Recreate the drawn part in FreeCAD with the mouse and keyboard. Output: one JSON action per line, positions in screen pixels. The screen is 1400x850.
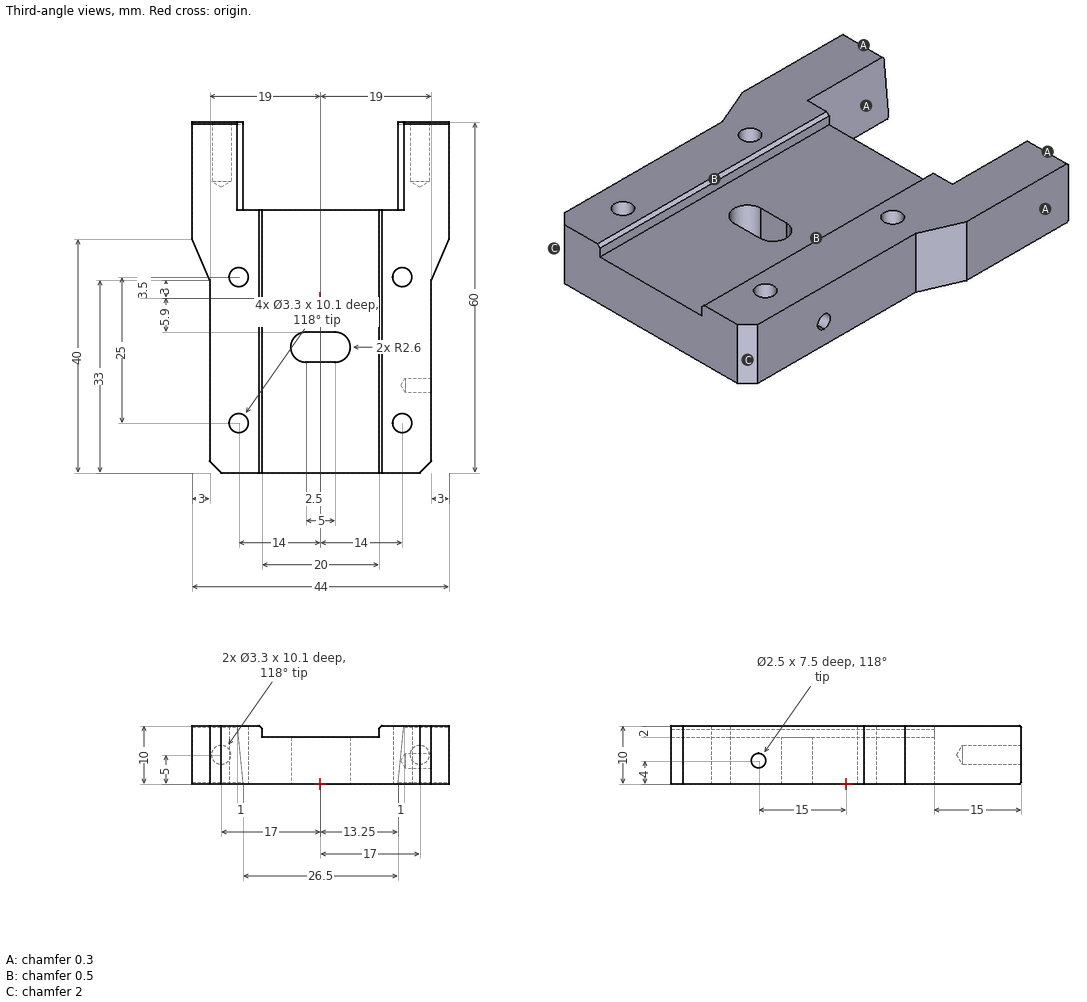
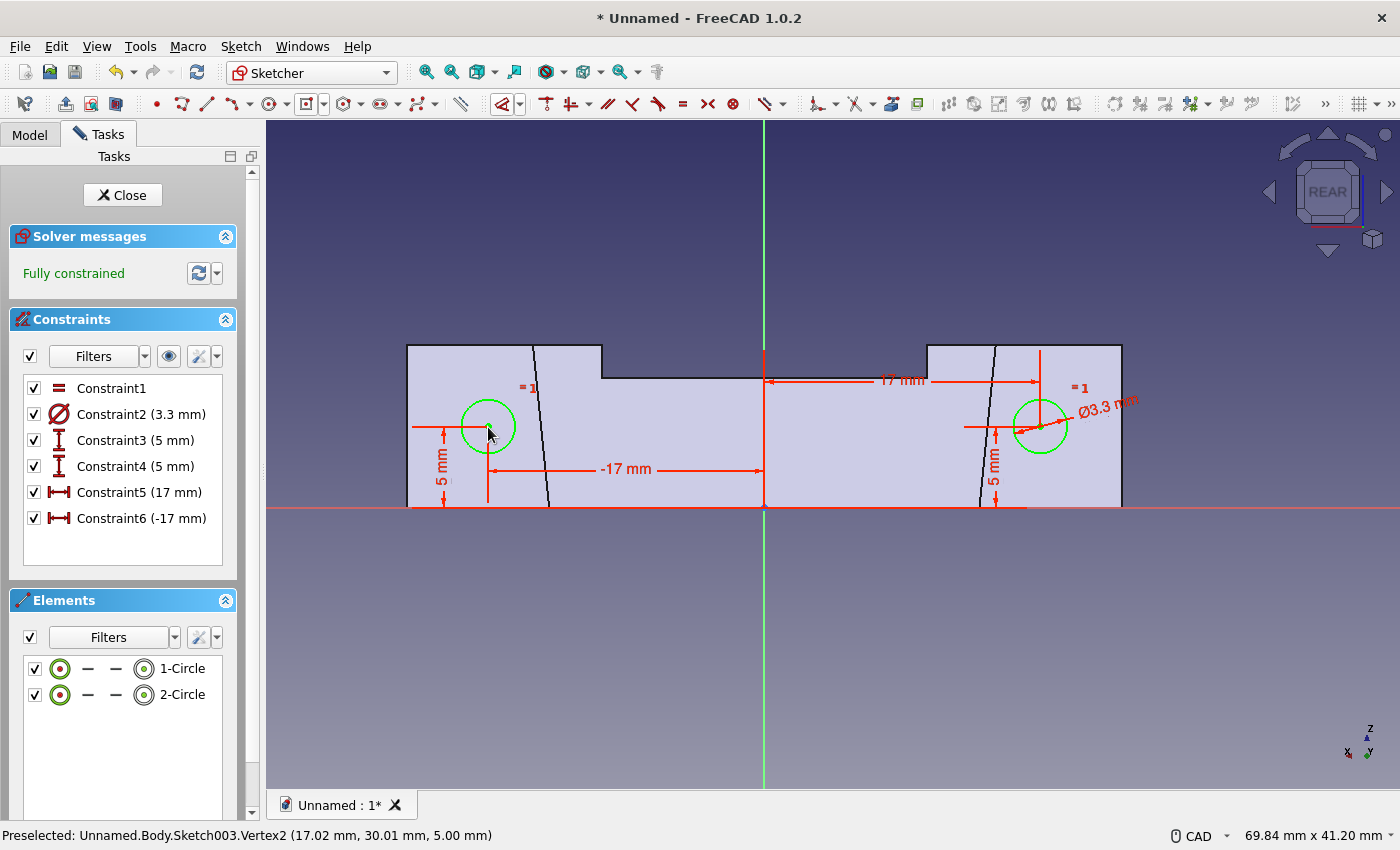
{"action": "left_click", "coordinate": [123, 195]}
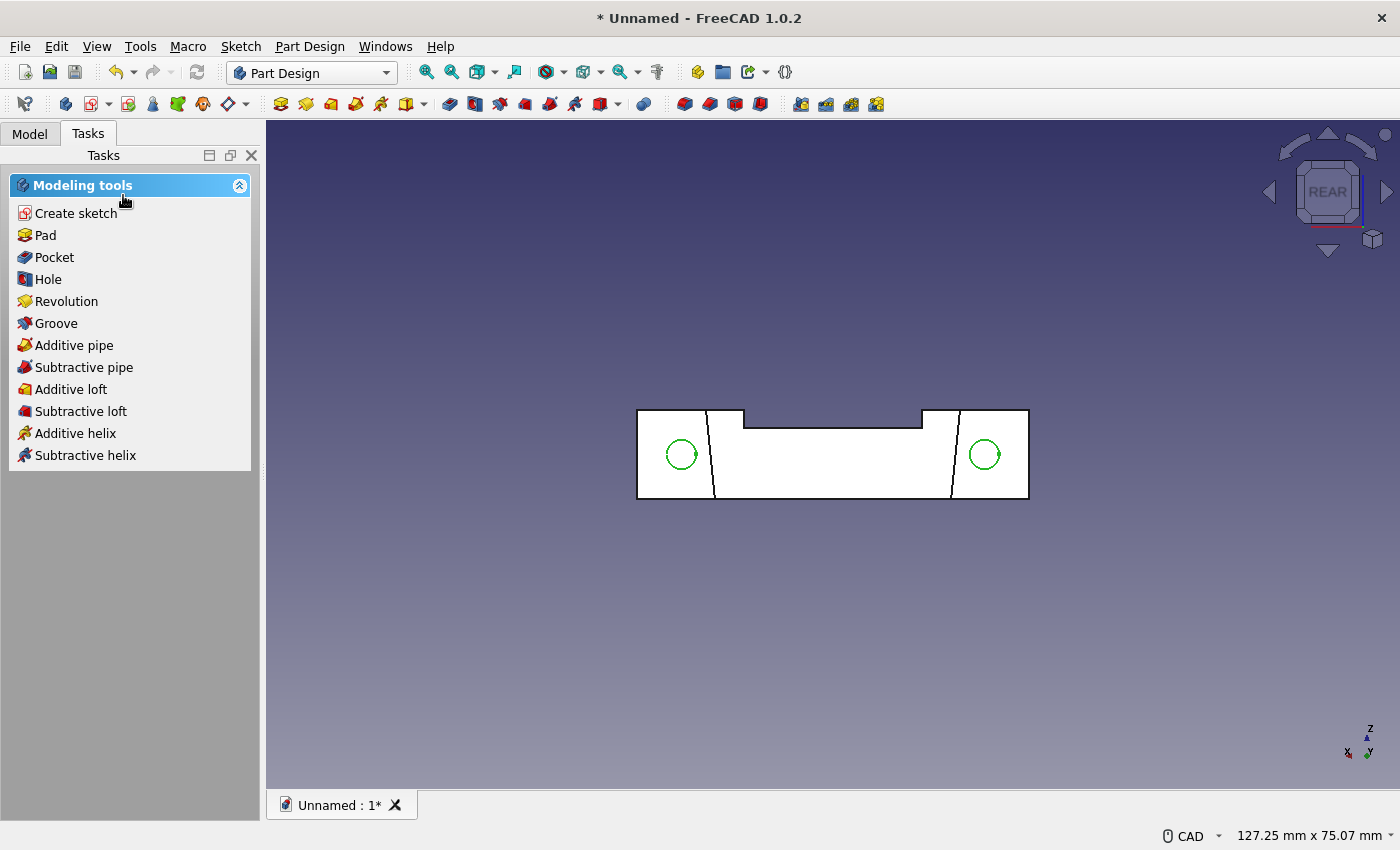
{"action": "left_click", "coordinate": [475, 104]}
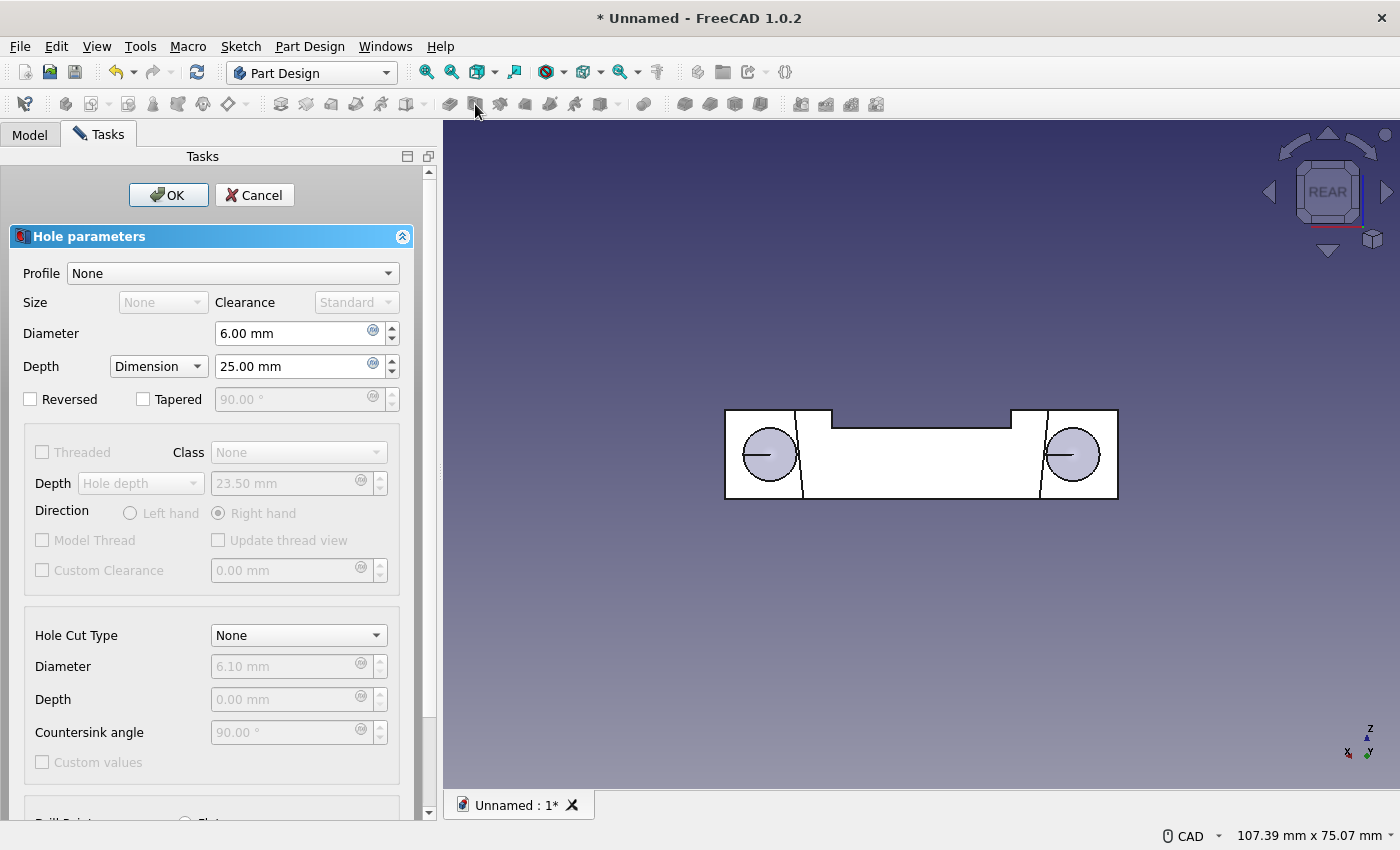
{"action": "triple_click", "coordinate": [300, 334]}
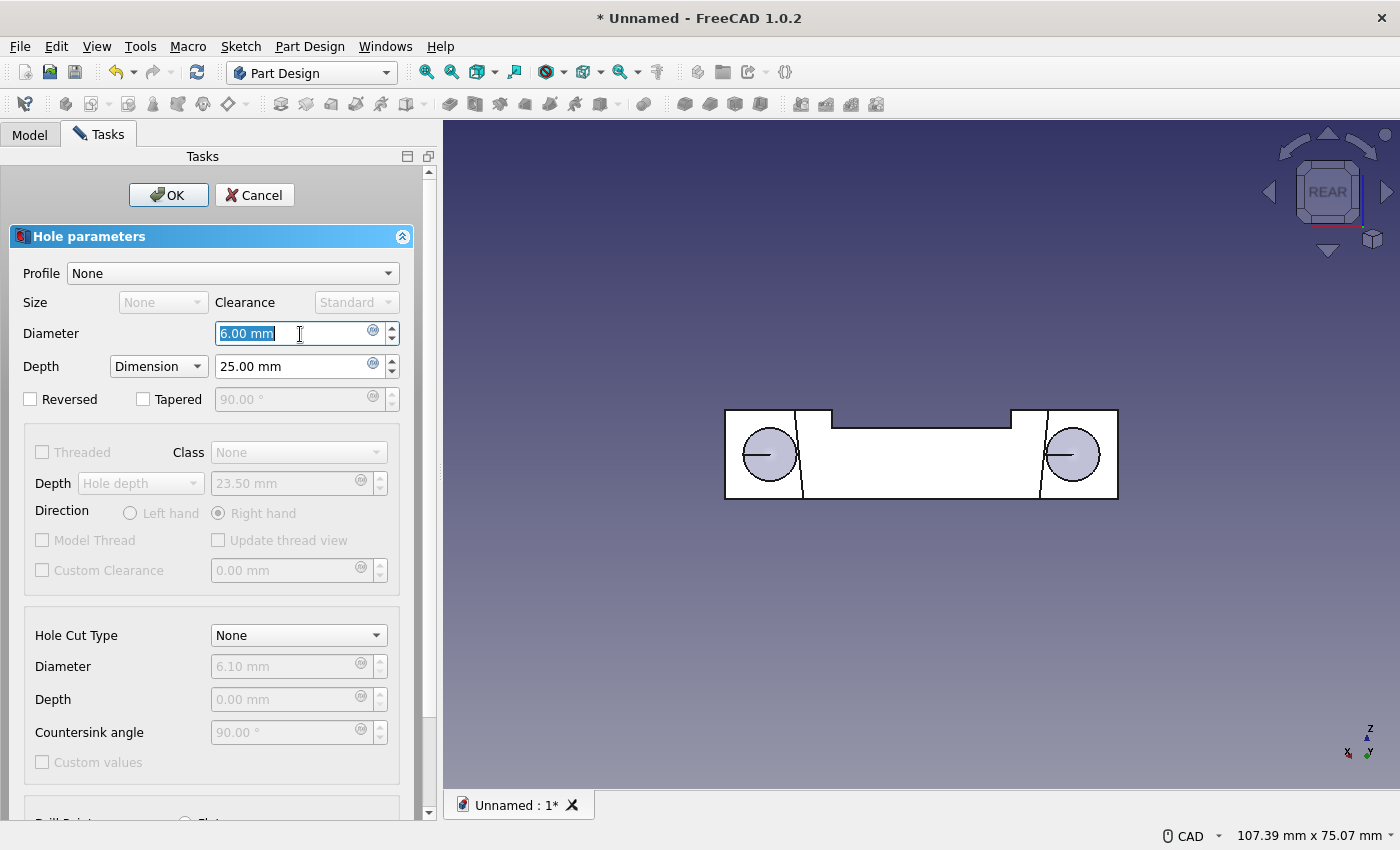
{"action": "type", "text": "3.3"}
{"action": "key", "text": "Tab"}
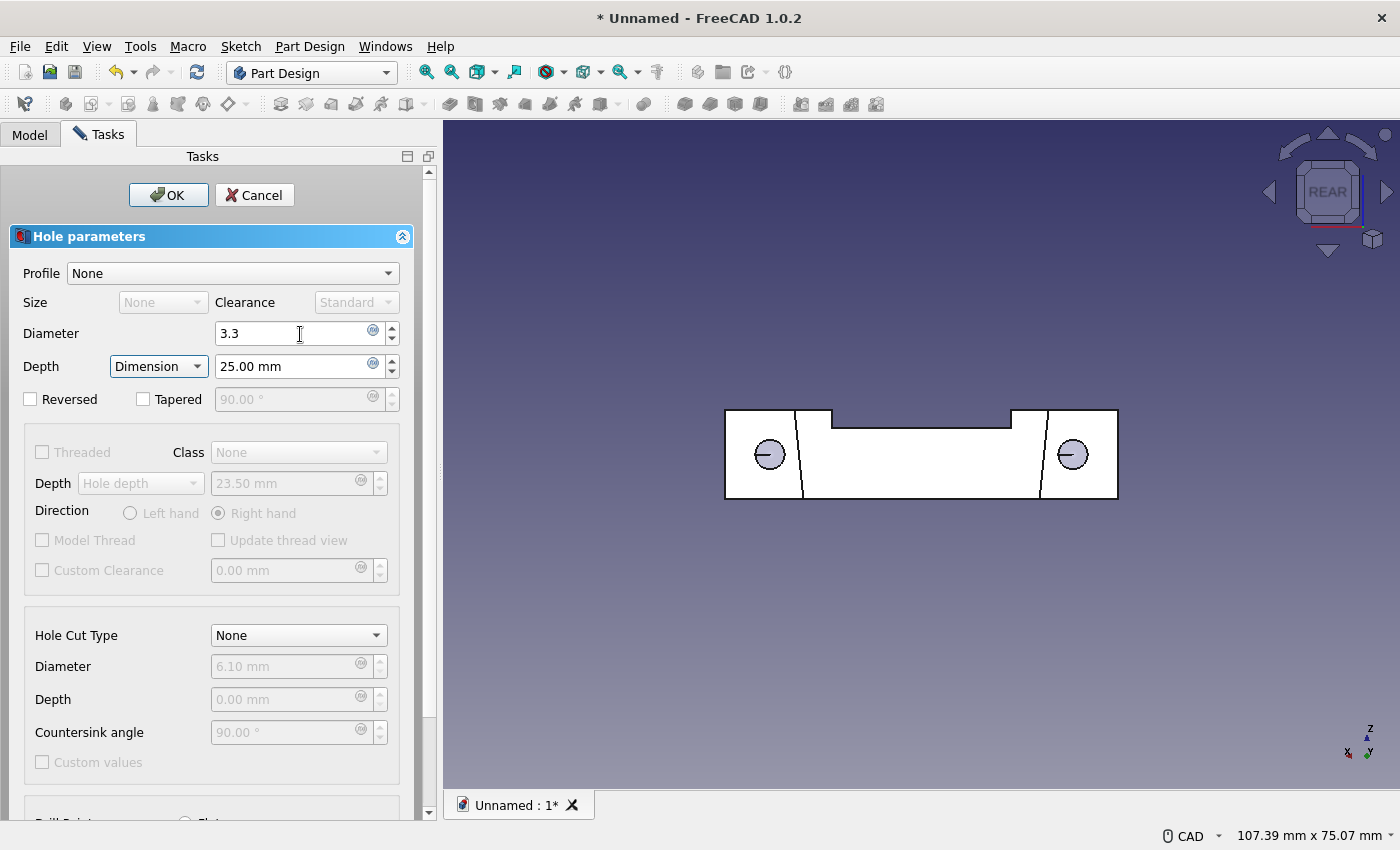
{"action": "triple_click", "coordinate": [300, 366]}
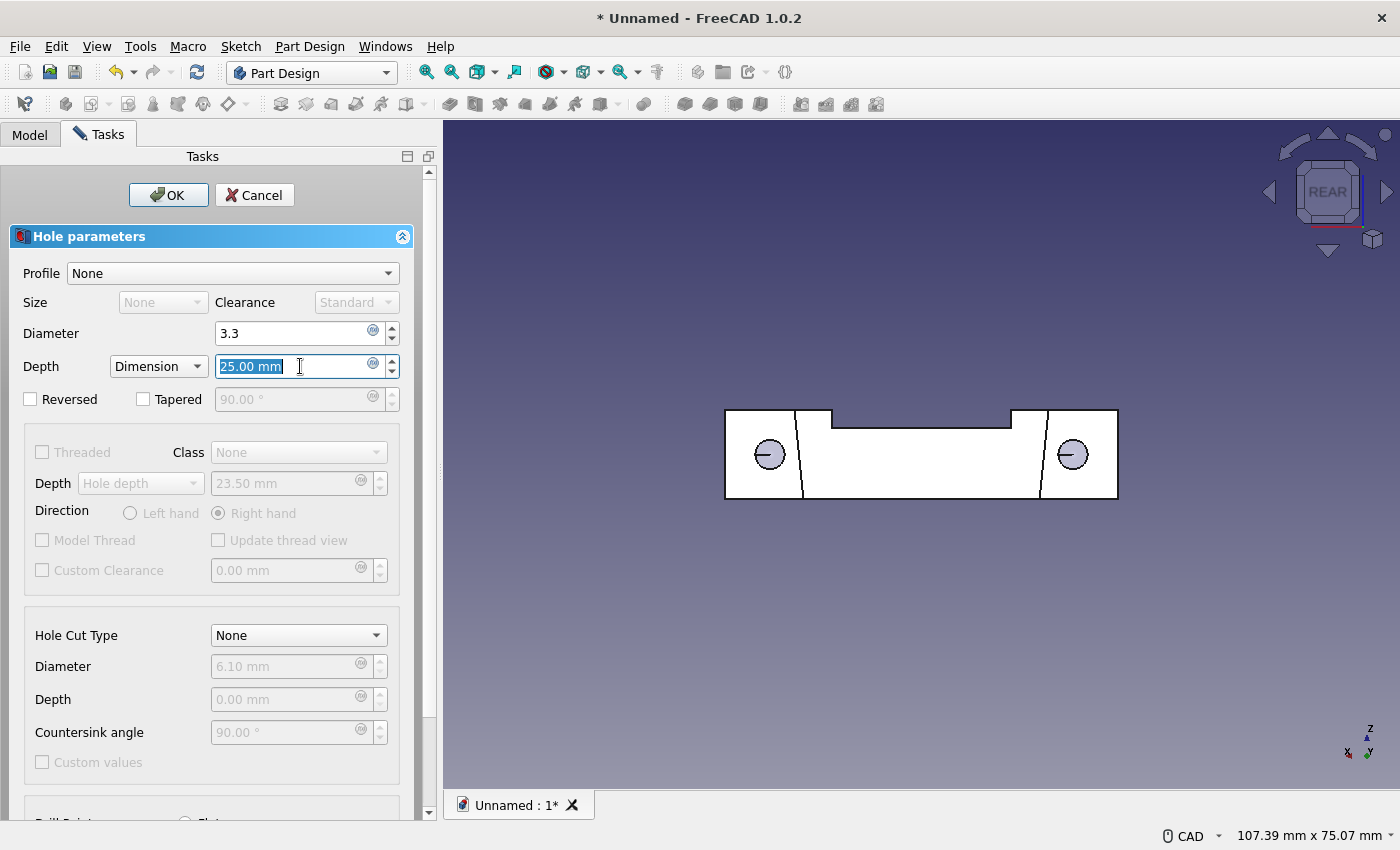
{"action": "type", "text": "10.1"}
{"action": "key", "text": "Tab"}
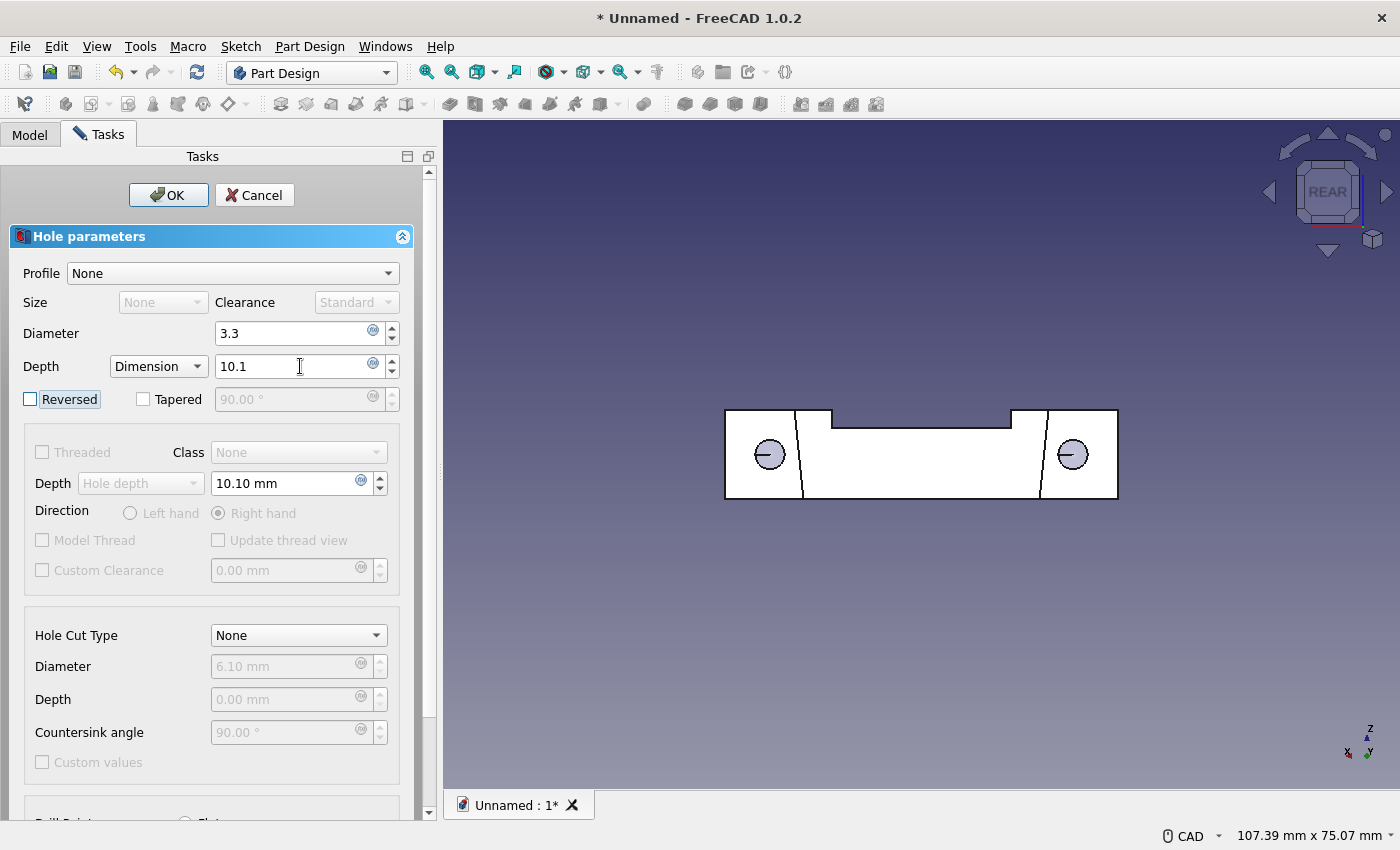
{"action": "left_click", "coordinate": [169, 195]}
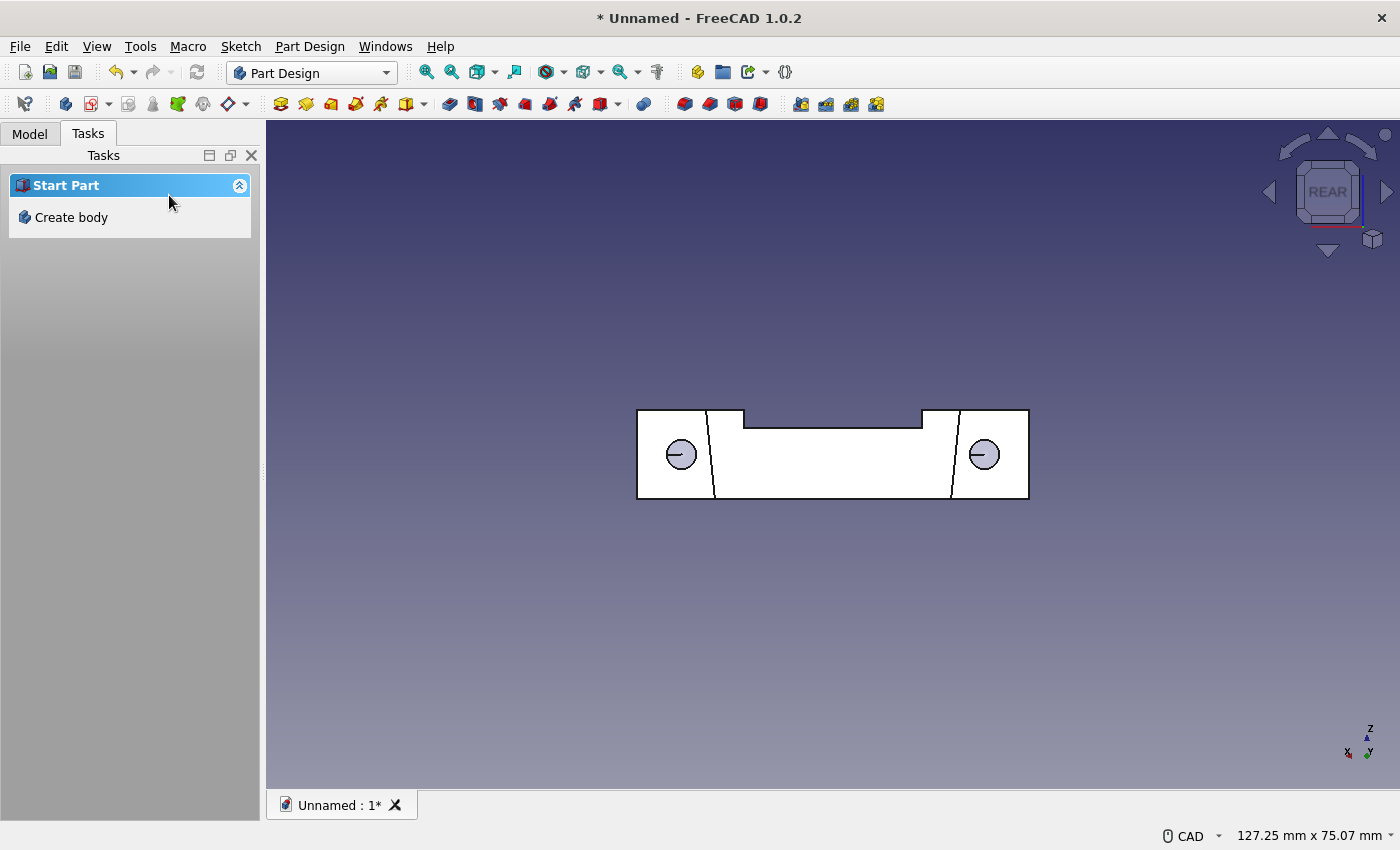
{"action": "left_click", "coordinate": [427, 72]}